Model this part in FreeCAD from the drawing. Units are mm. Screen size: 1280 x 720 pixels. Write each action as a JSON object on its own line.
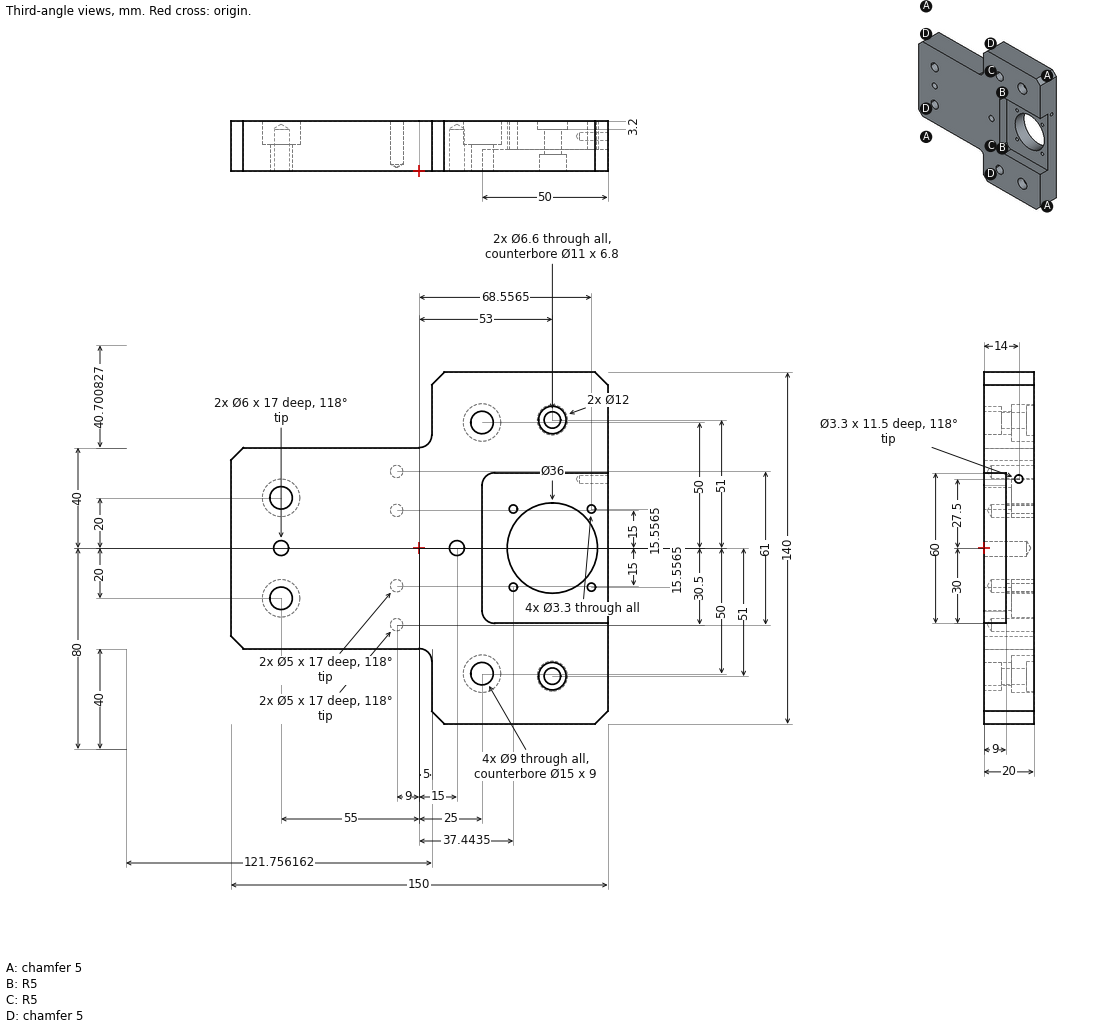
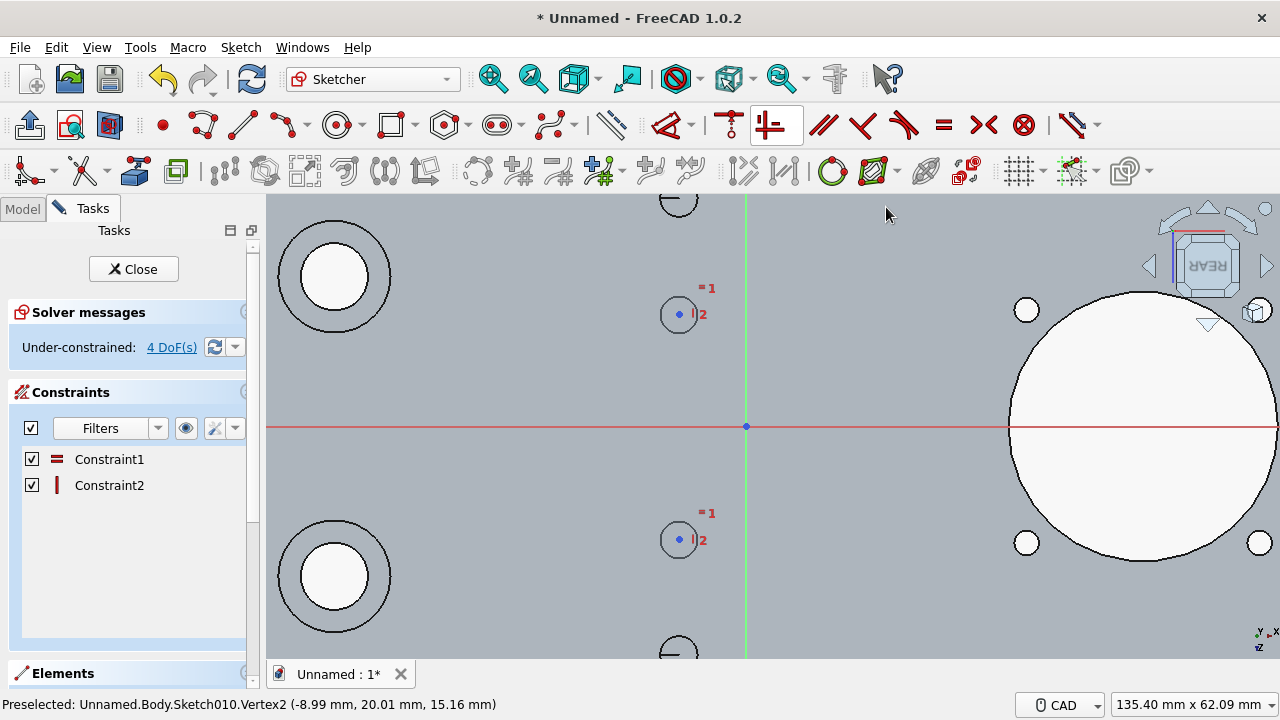
{"action": "left_click", "coordinate": [666, 126]}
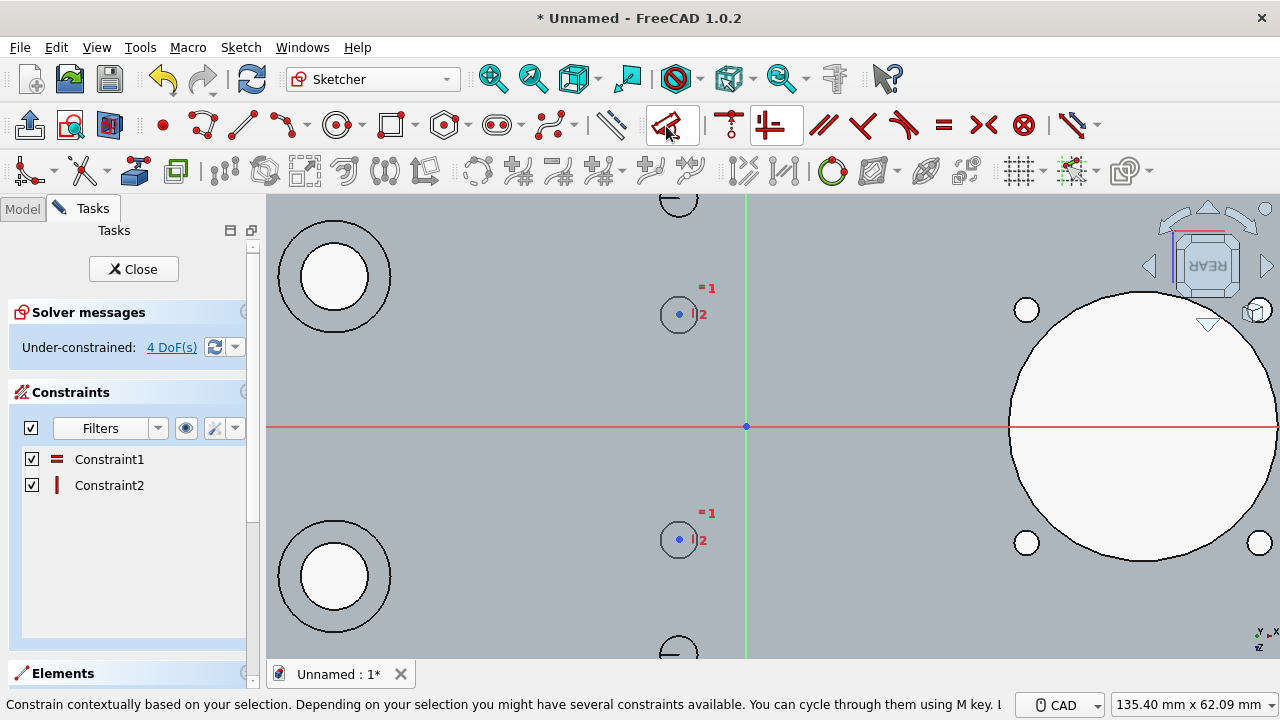
{"action": "left_click", "coordinate": [692, 302]}
{"action": "left_click", "coordinate": [715, 279]}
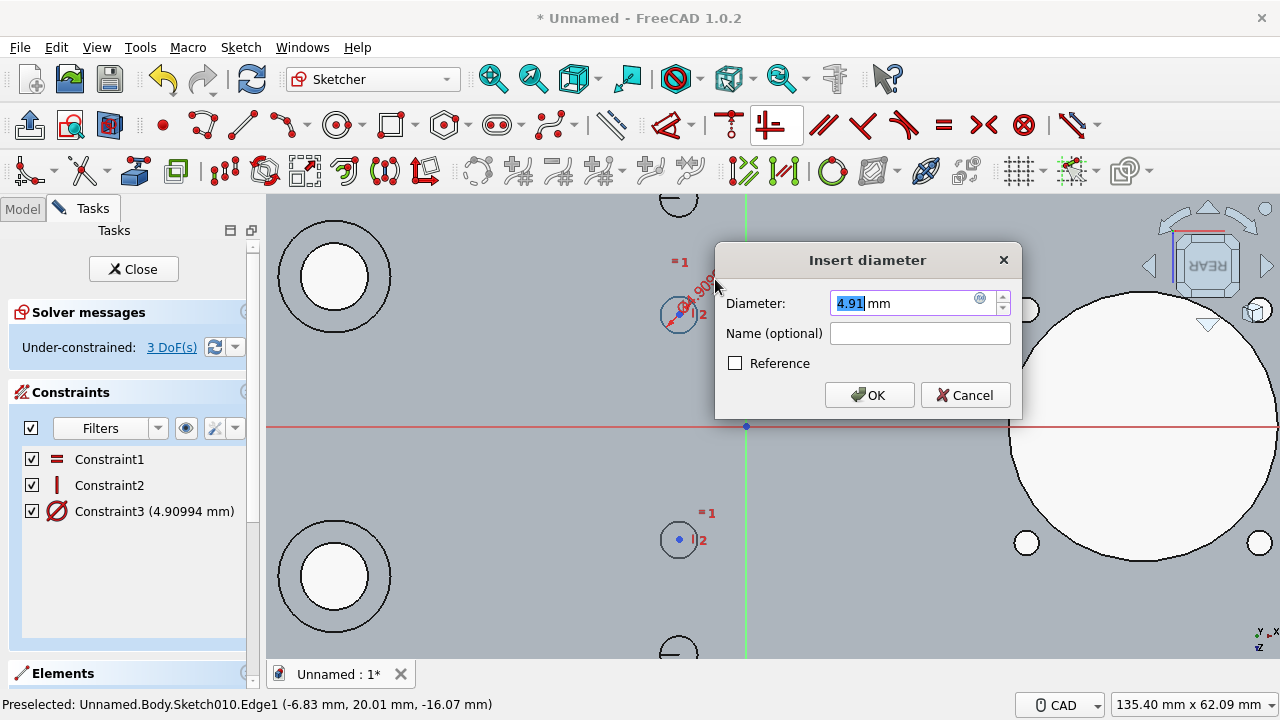
{"action": "type", "text": "5"}
{"action": "key", "text": "Return"}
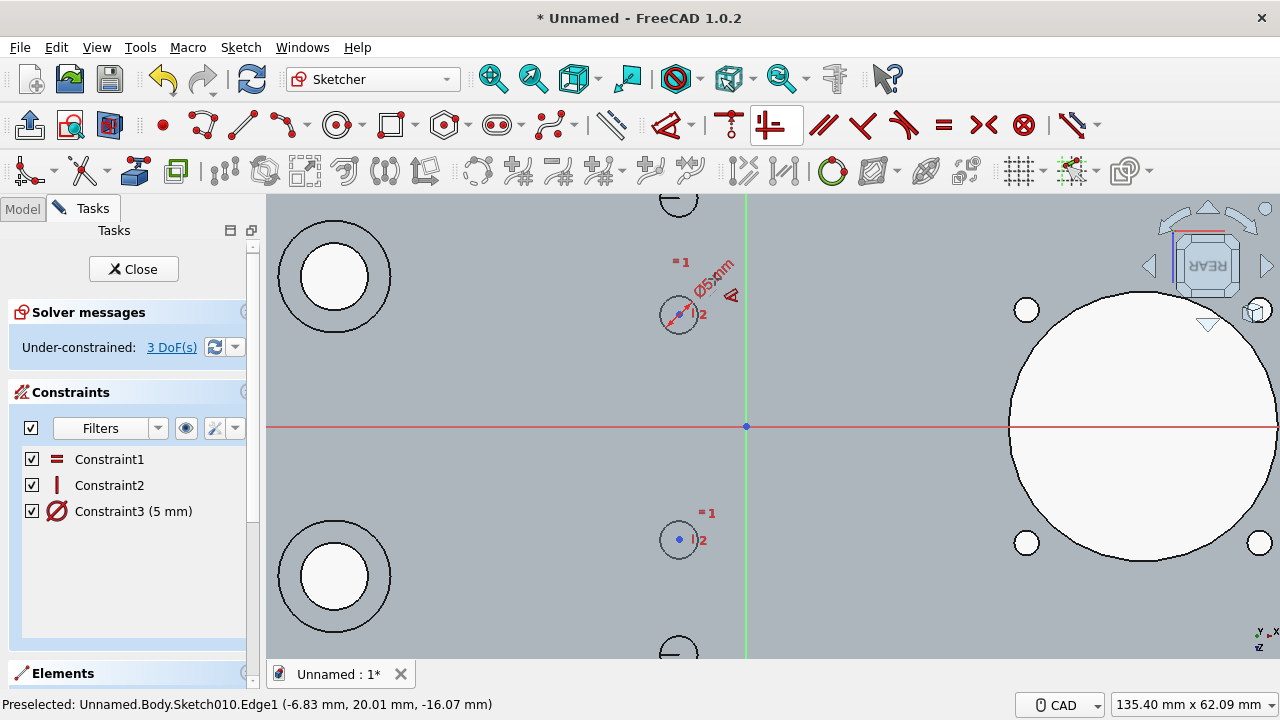
{"action": "left_click", "coordinate": [679, 315]}
{"action": "left_click", "coordinate": [713, 460]}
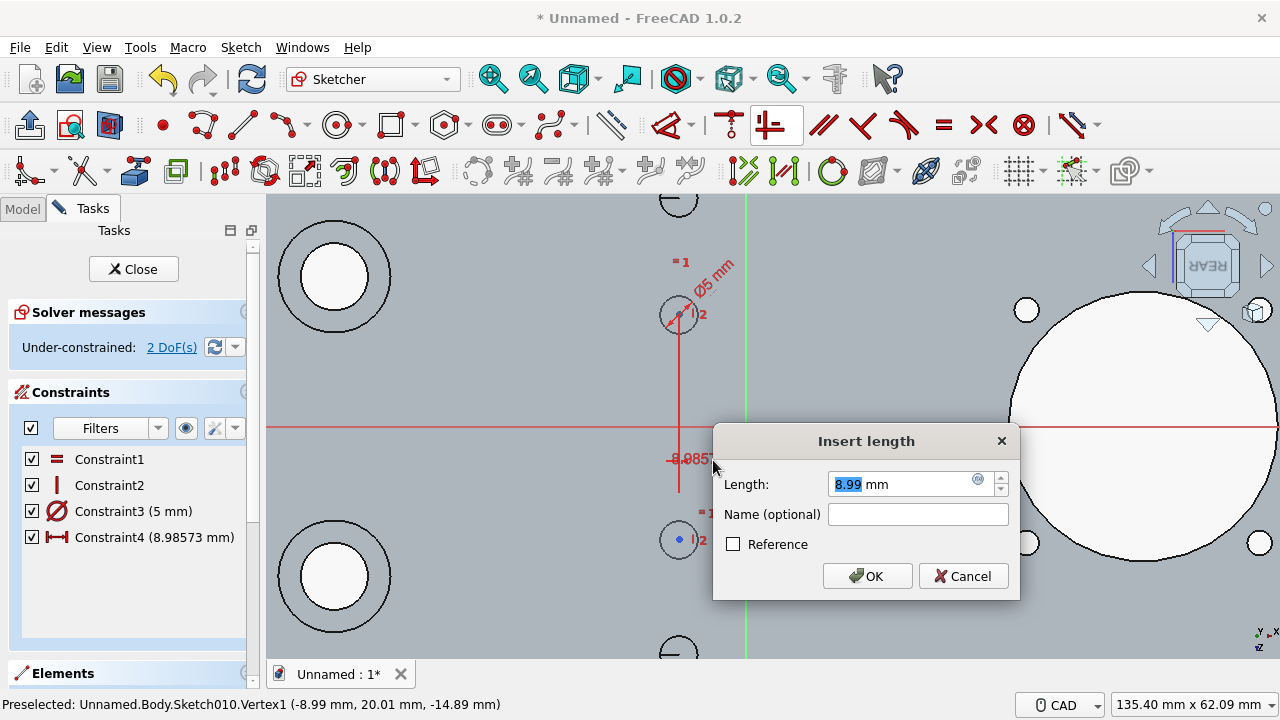
{"action": "type", "text": "9"}
{"action": "key", "text": "Return"}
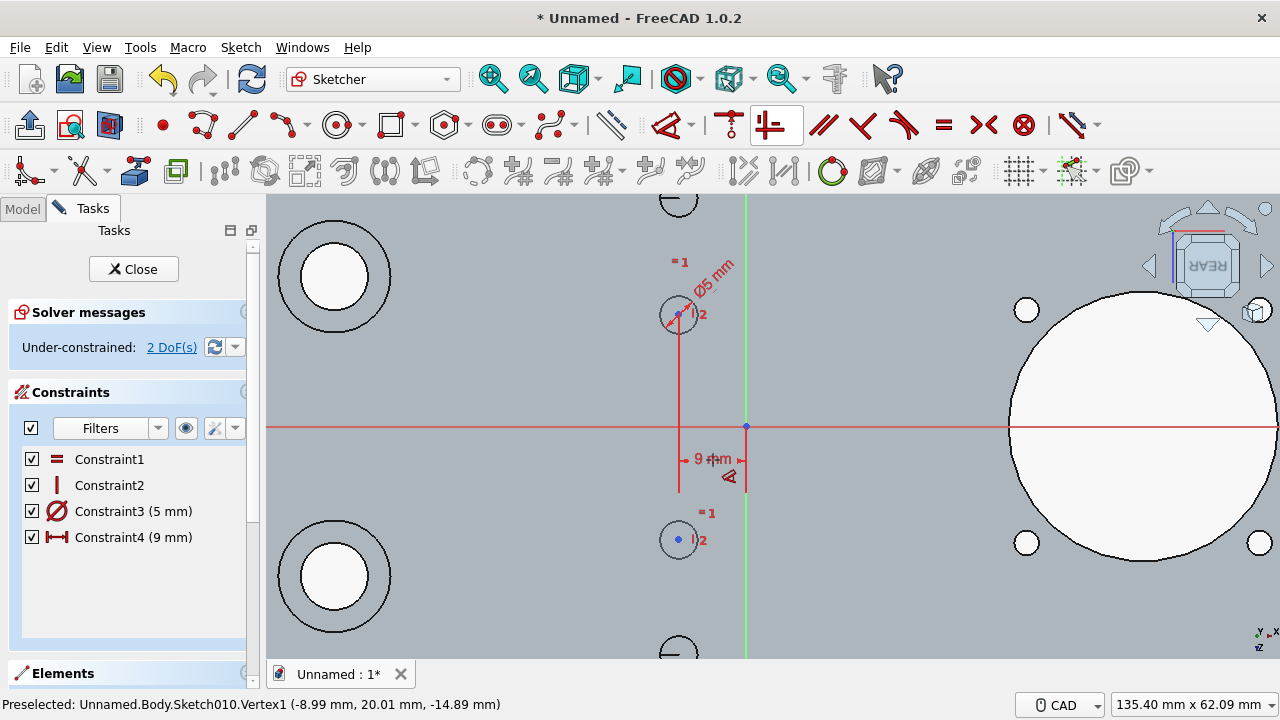
{"action": "left_click", "coordinate": [679, 315]}
{"action": "left_click", "coordinate": [780, 371]}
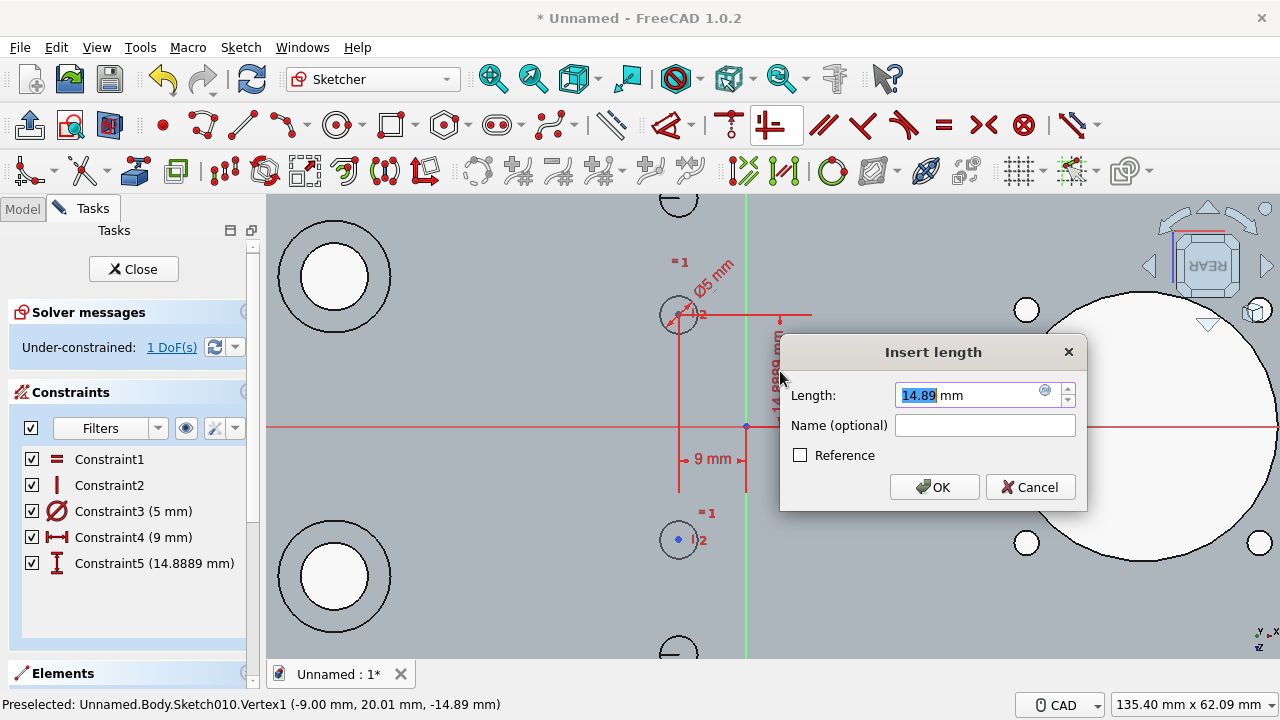
{"action": "type", "text": "15"}
{"action": "key", "text": "Return"}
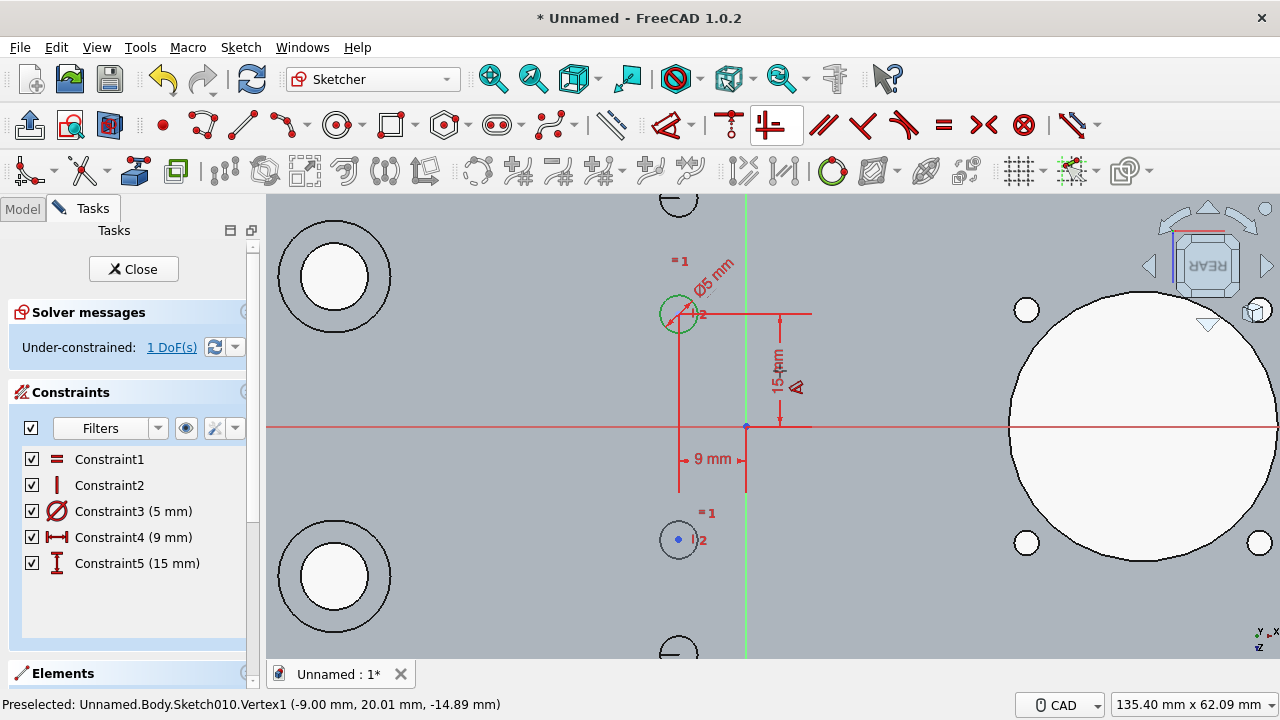
{"action": "left_click", "coordinate": [679, 540]}
{"action": "left_click", "coordinate": [780, 483]}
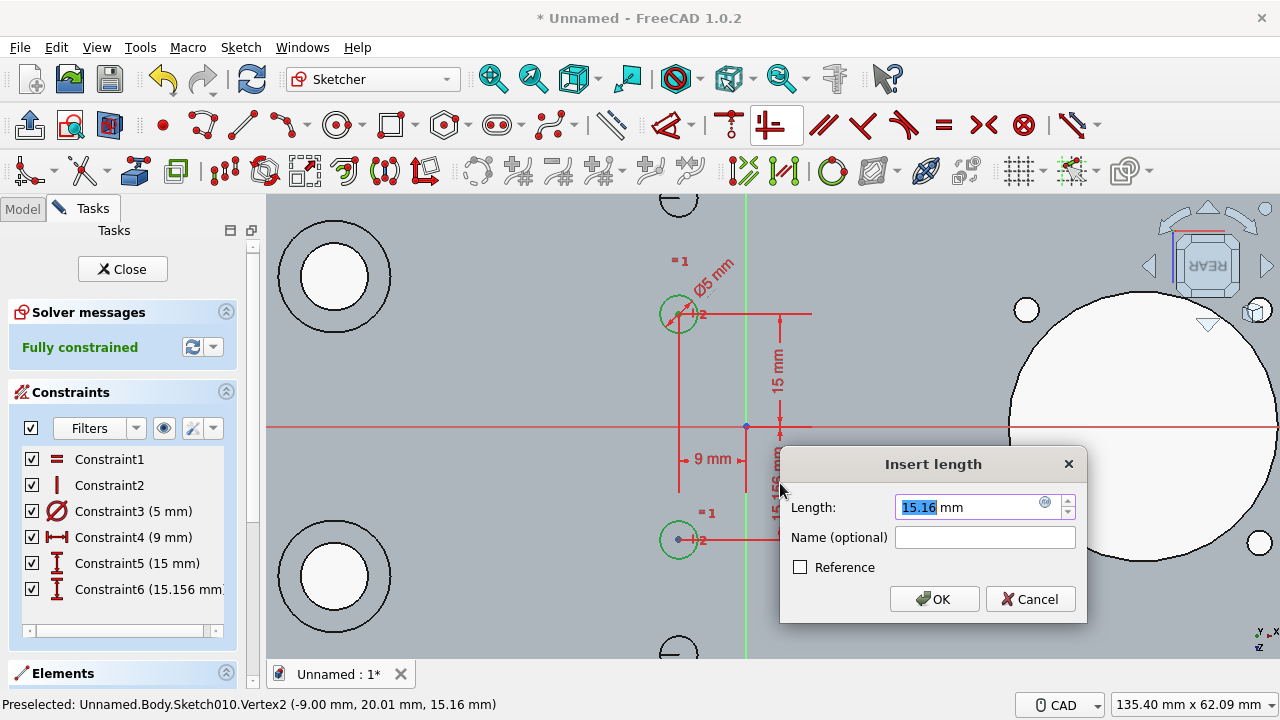
{"action": "type", "text": "15"}
{"action": "key", "text": "Return"}
{"action": "key", "text": "Escape"}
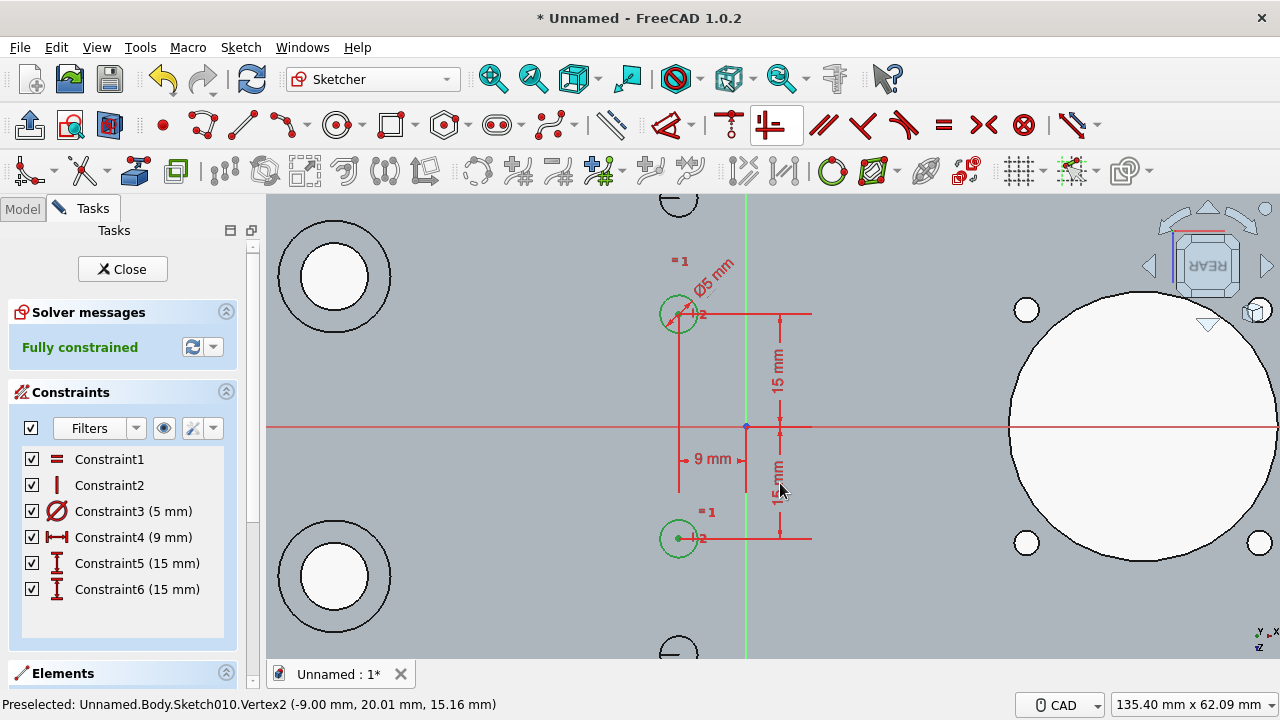
{"action": "left_click", "coordinate": [123, 269]}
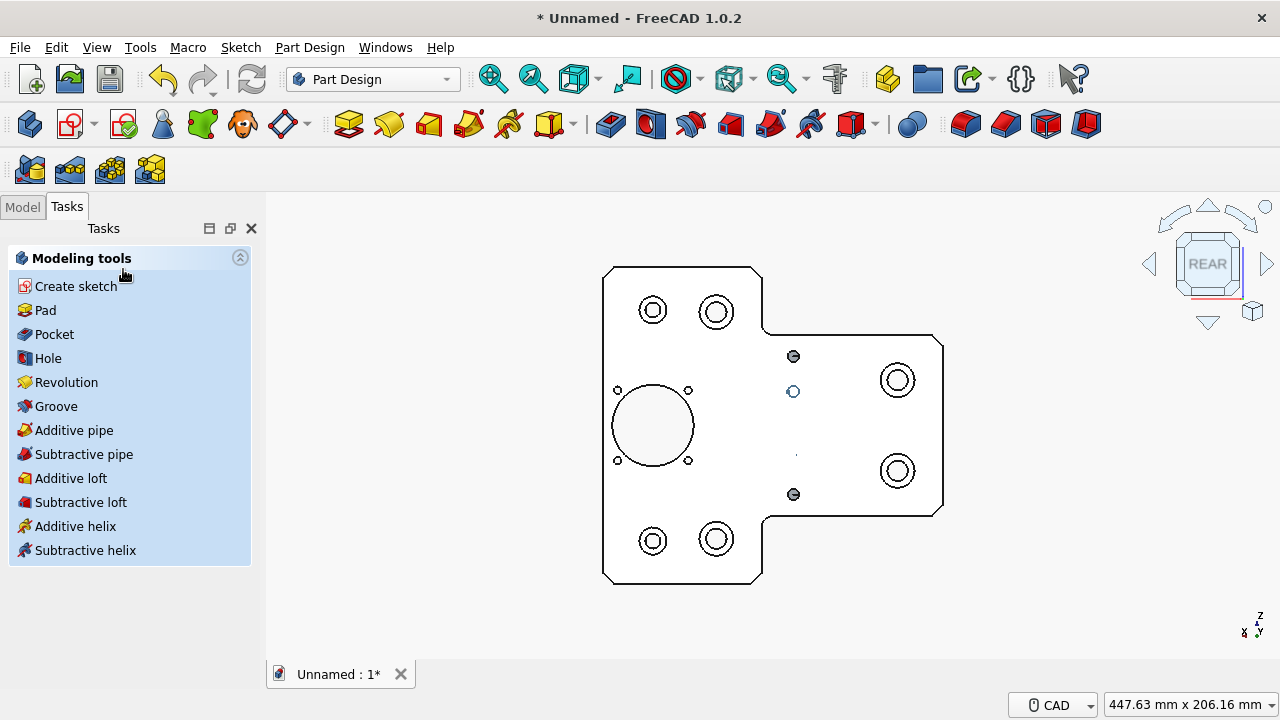
{"action": "left_click", "coordinate": [652, 124]}